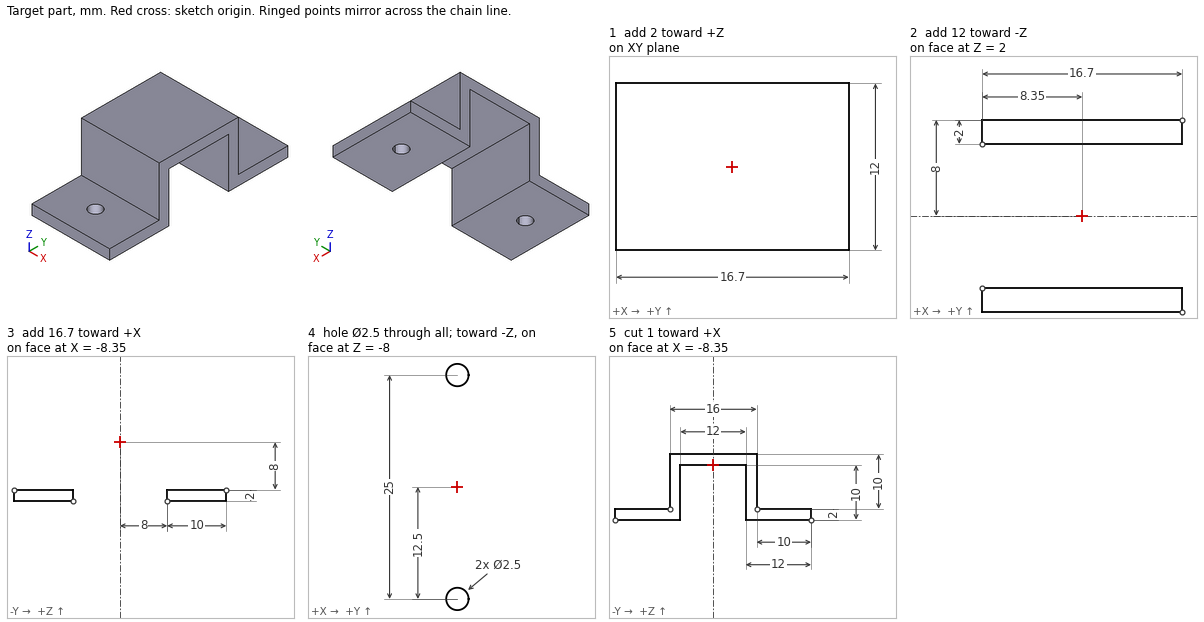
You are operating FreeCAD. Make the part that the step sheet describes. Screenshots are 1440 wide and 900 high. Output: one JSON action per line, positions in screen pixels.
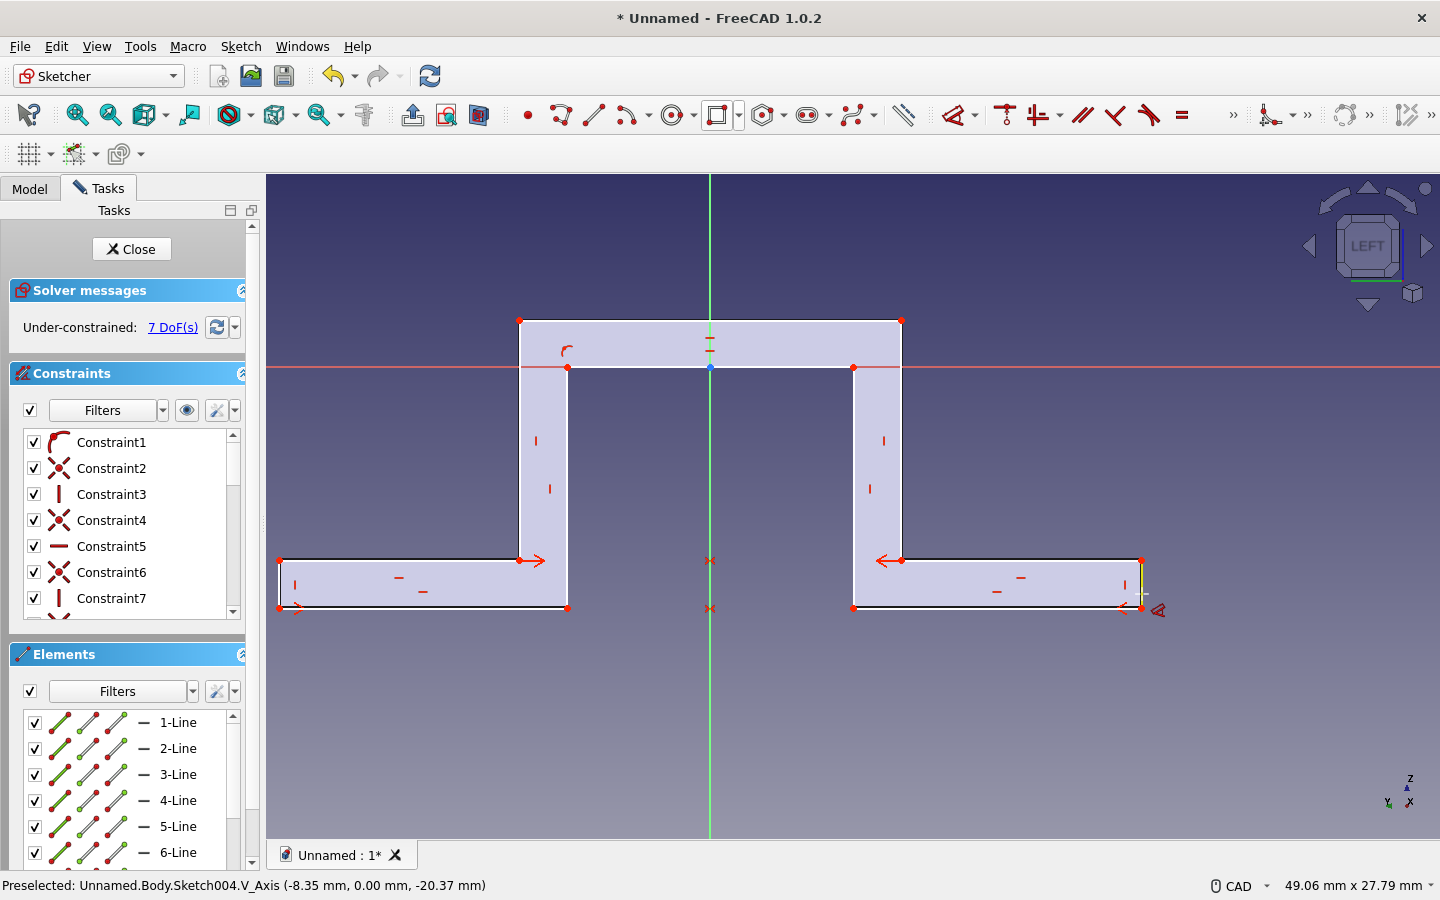
{"action": "left_click", "coordinate": [1142, 594]}
{"action": "left_click", "coordinate": [1176, 585]}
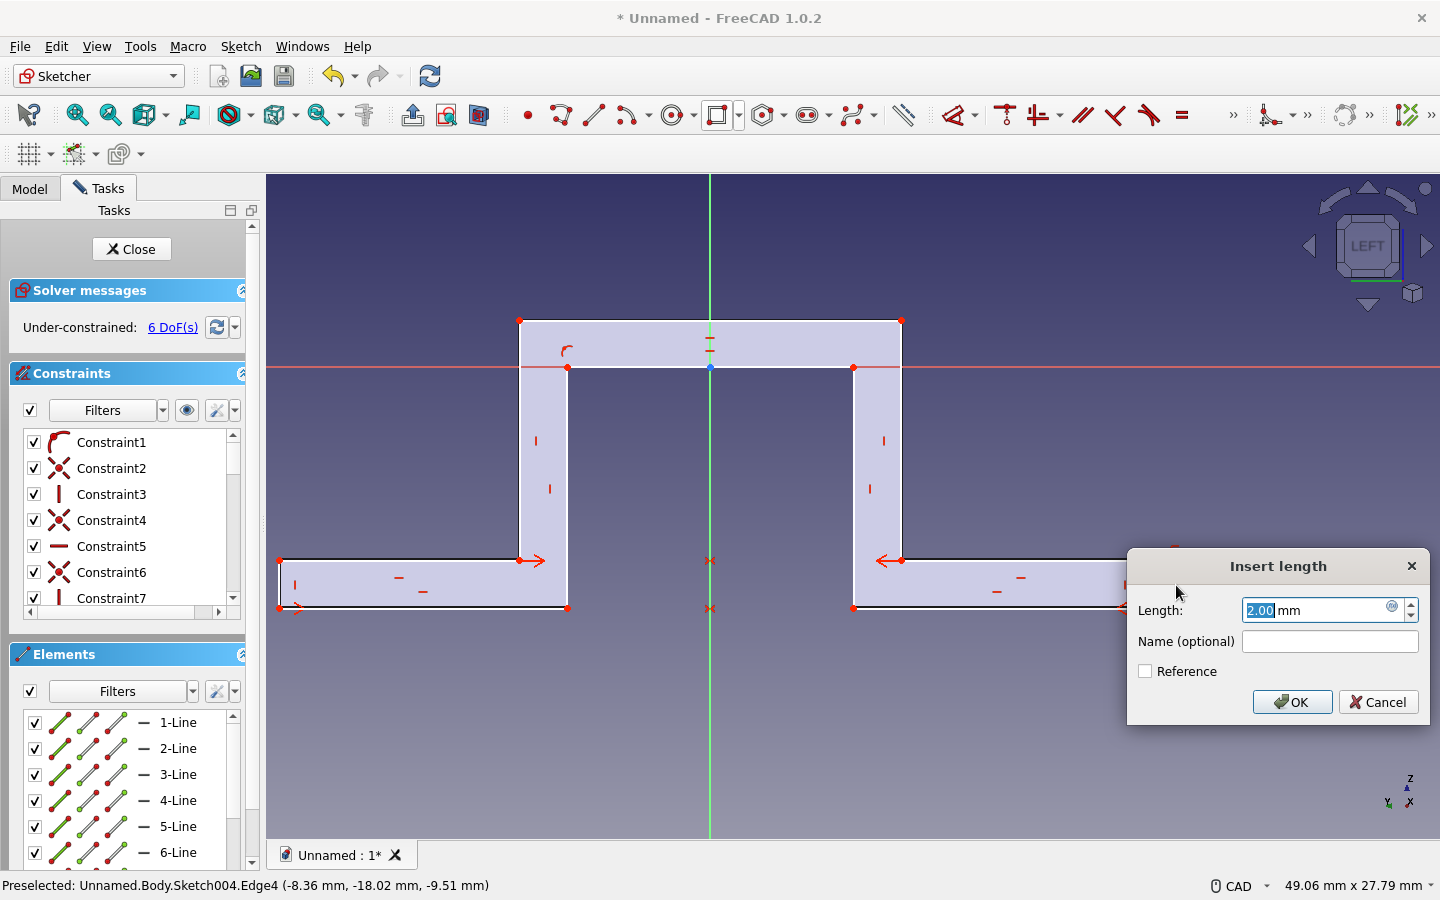
{"action": "type", "text": "2"}
{"action": "key", "text": "Return"}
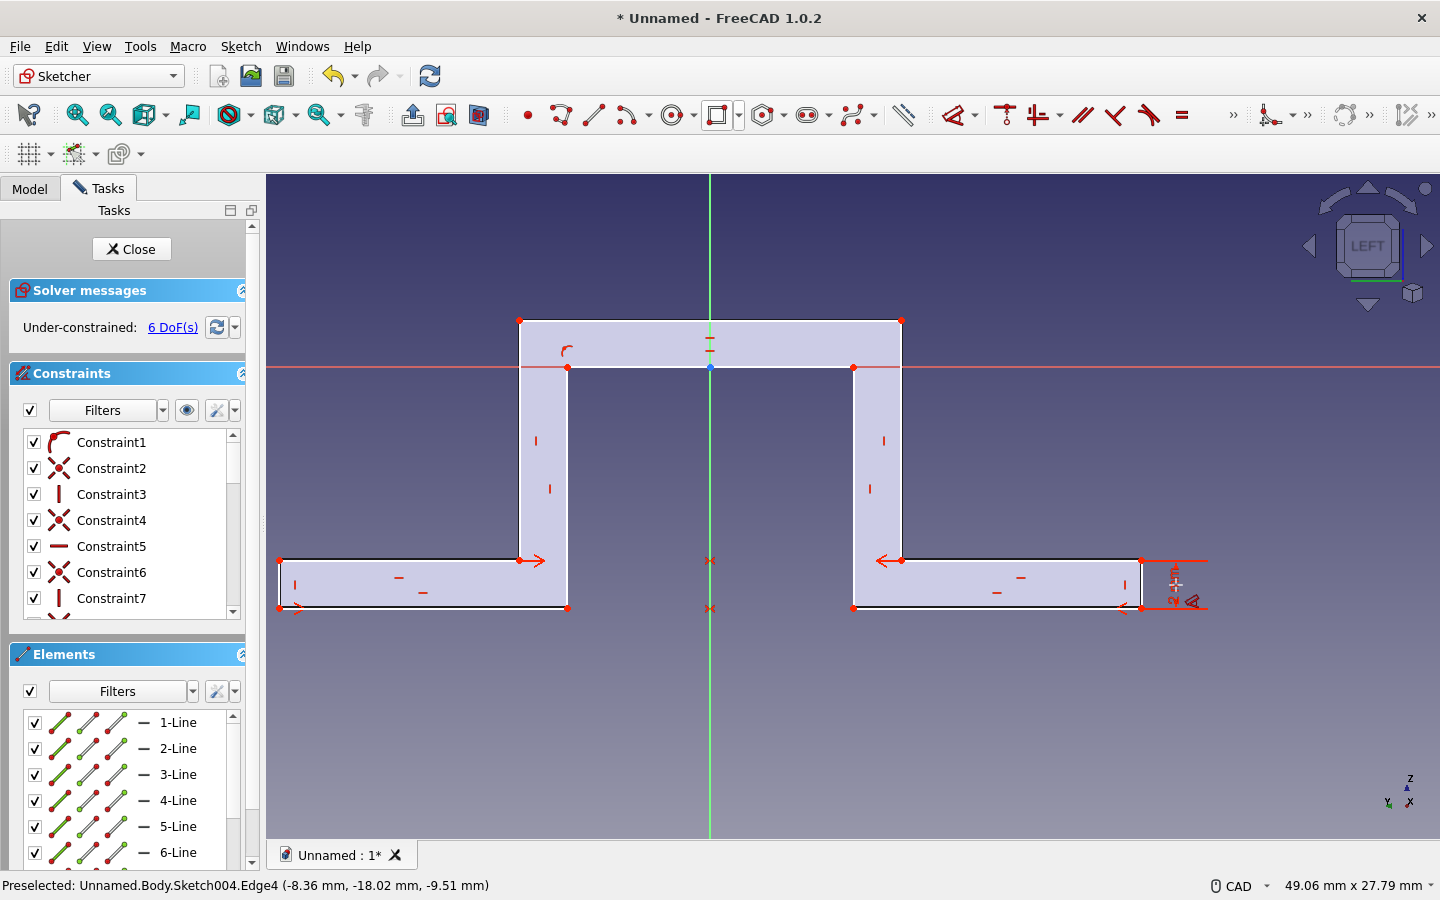
{"action": "left_click", "coordinate": [653, 367]}
{"action": "left_click", "coordinate": [645, 401]}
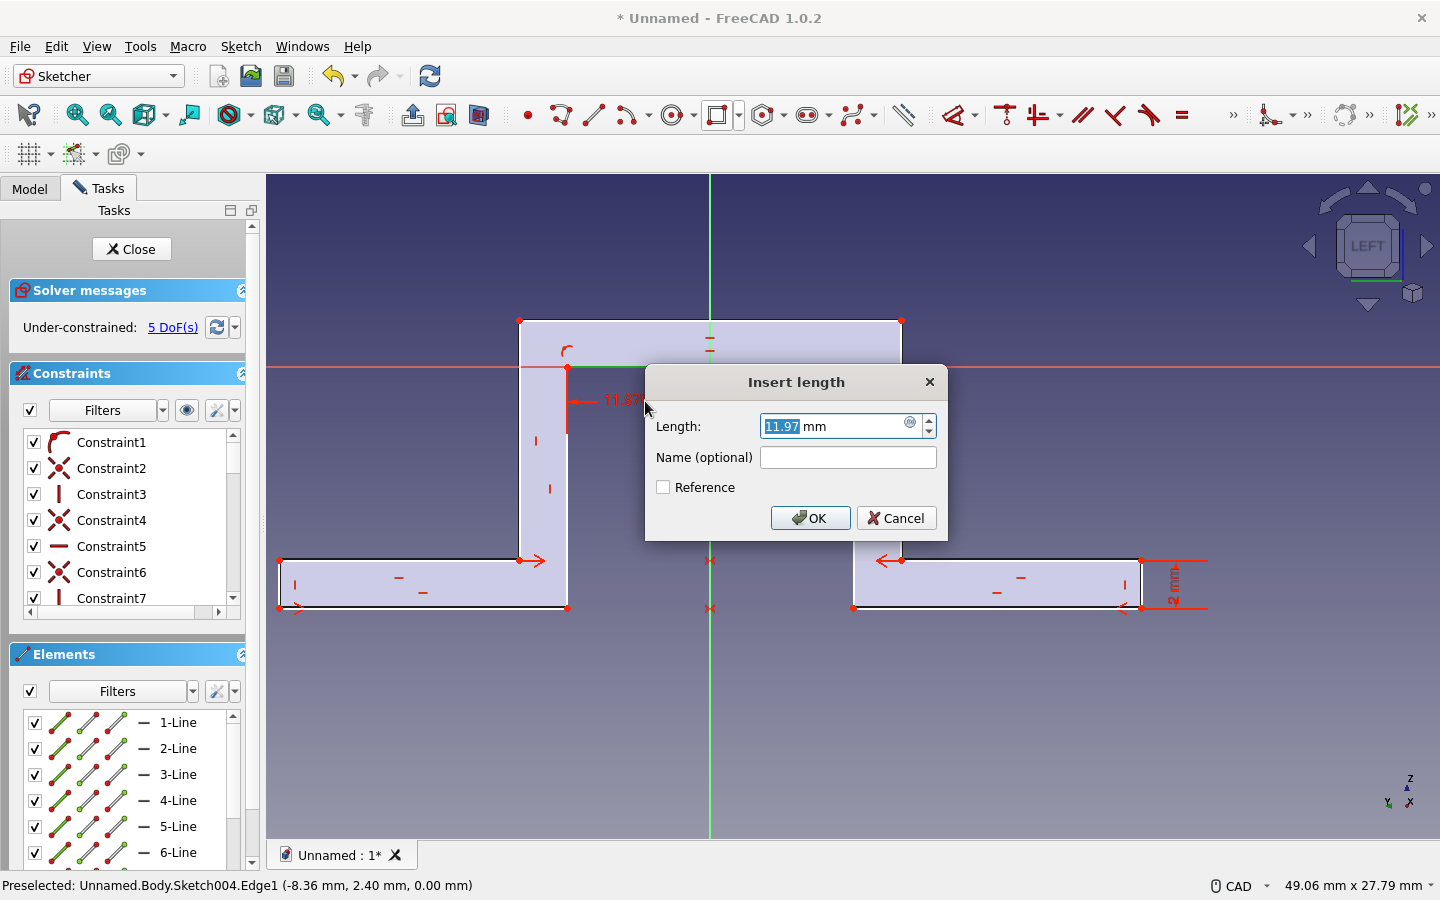
{"action": "type", "text": "12"}
{"action": "key", "text": "Return"}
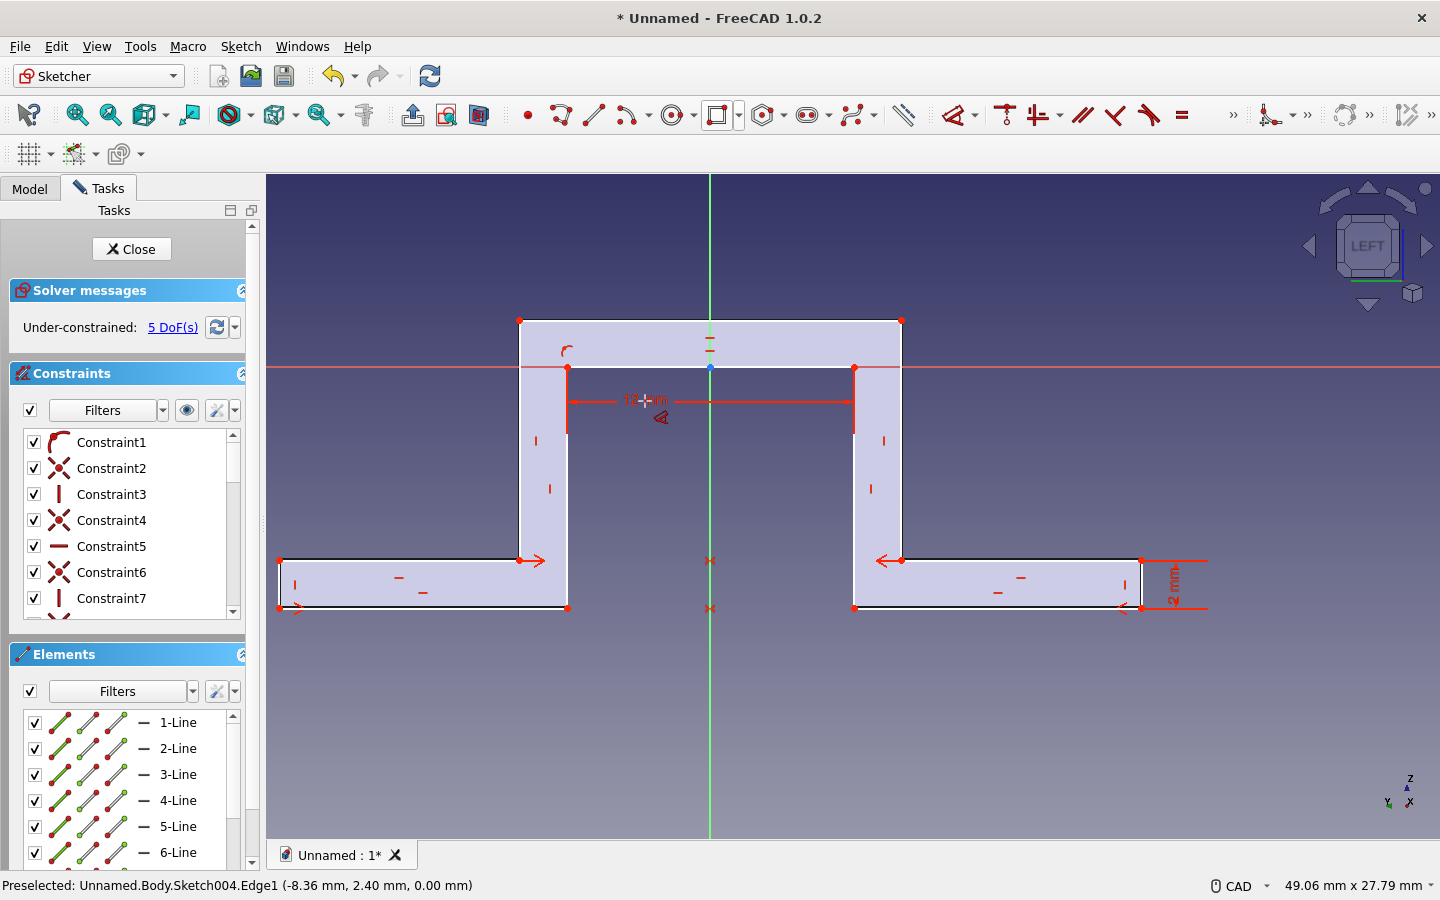
{"action": "left_click", "coordinate": [854, 440]}
{"action": "left_click", "coordinate": [888, 488]}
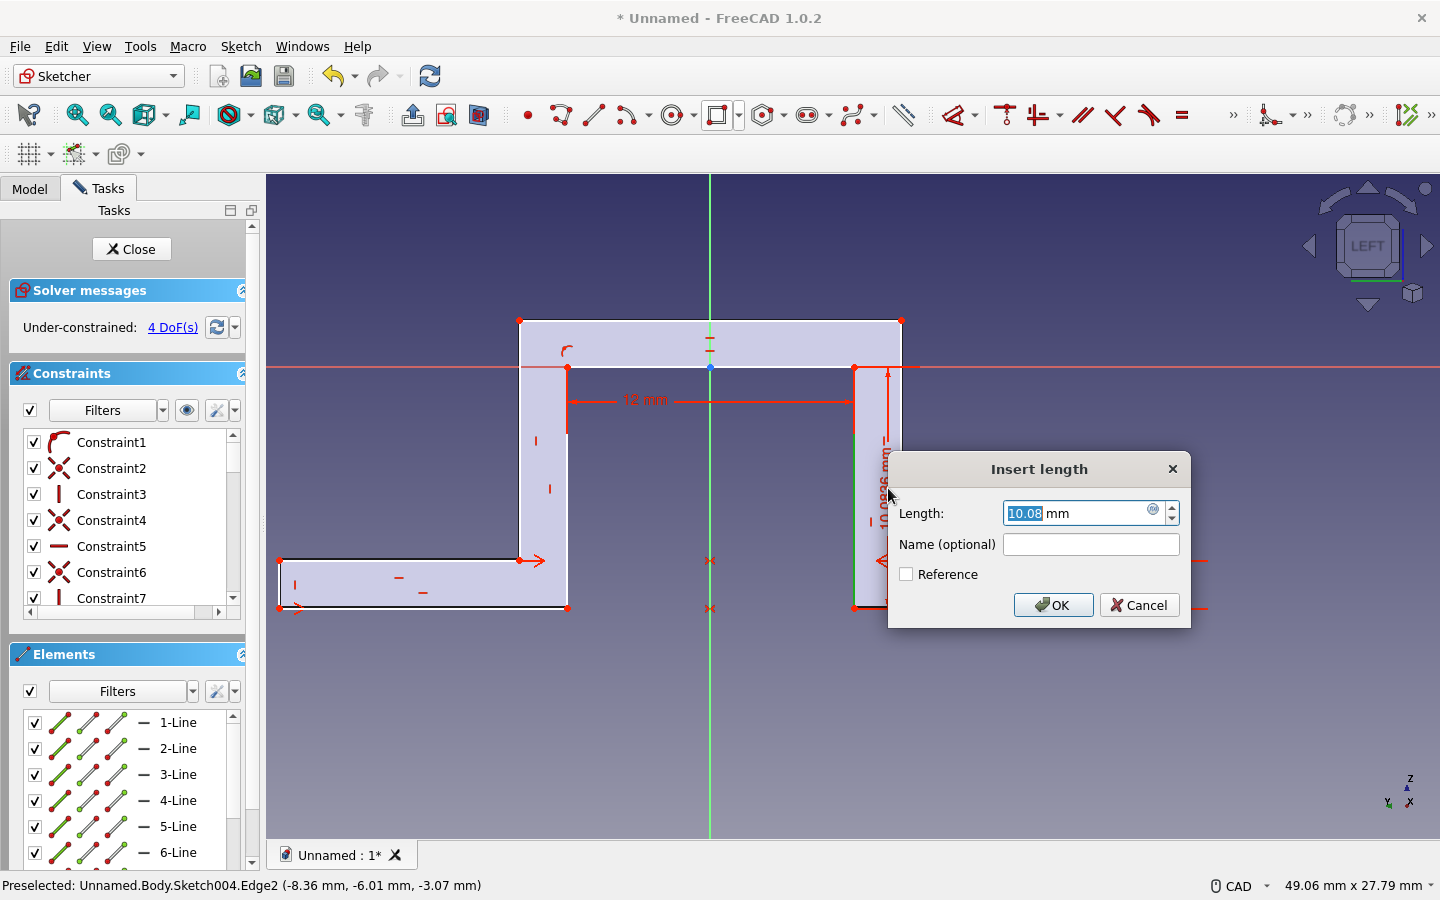
{"action": "type", "text": "10"}
{"action": "key", "text": "Return"}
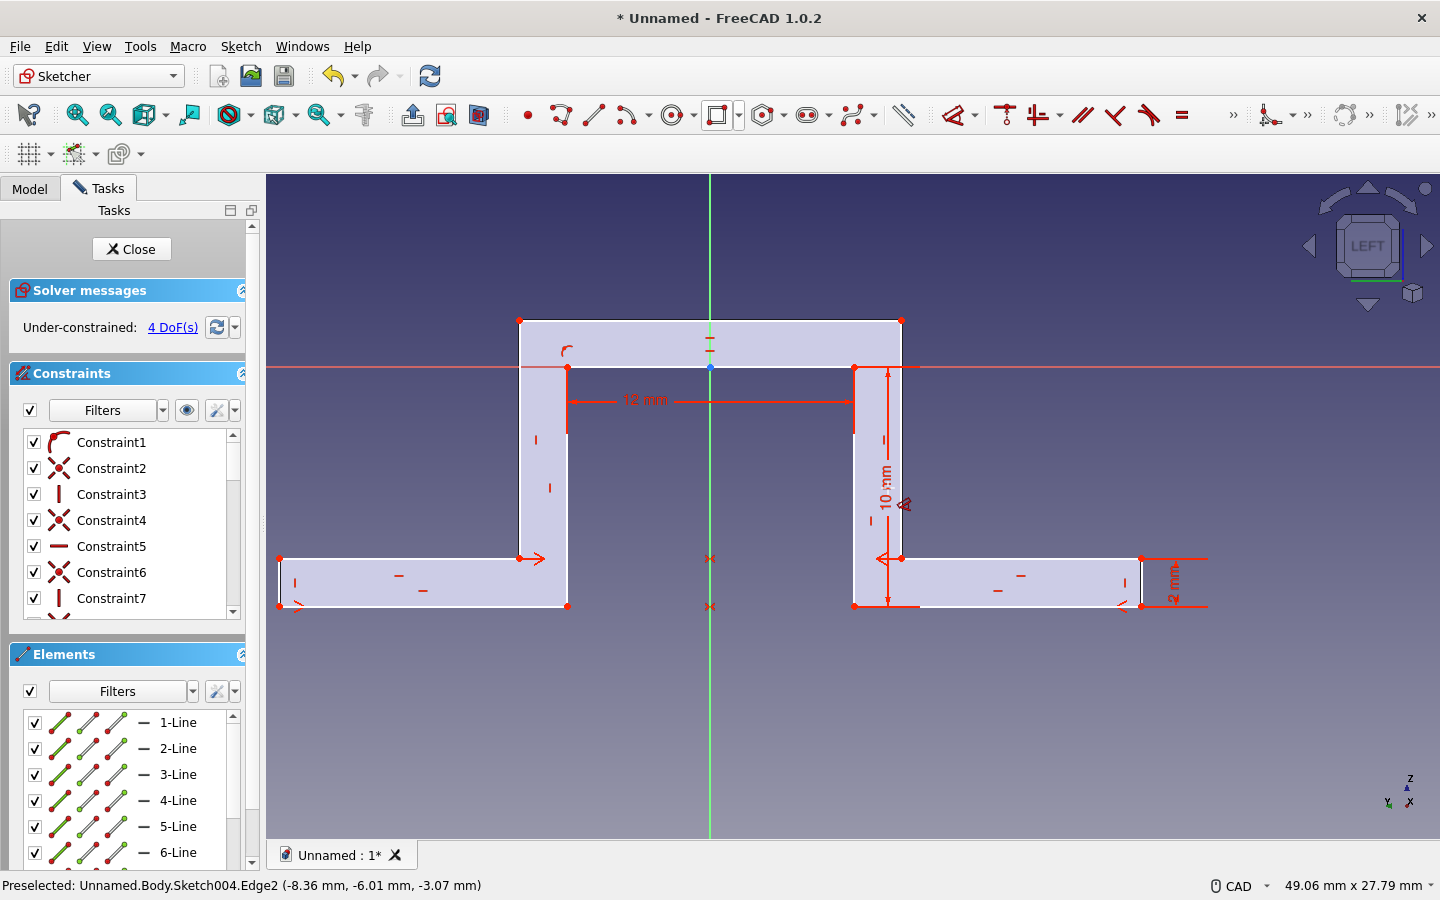
{"action": "left_click", "coordinate": [941, 607]}
{"action": "left_click", "coordinate": [998, 641]}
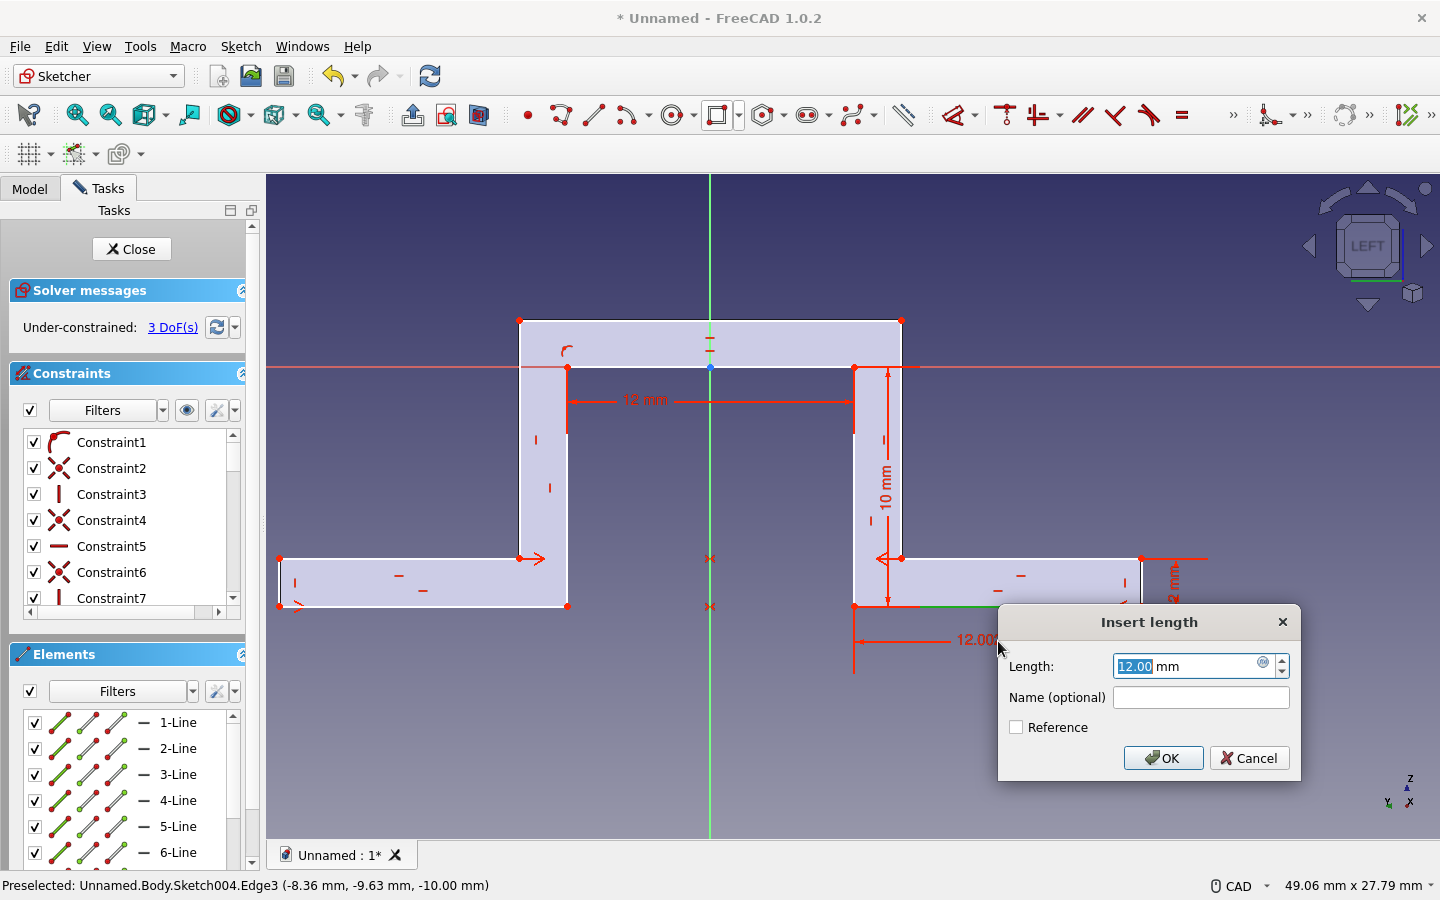
{"action": "type", "text": "12"}
{"action": "key", "text": "Return"}